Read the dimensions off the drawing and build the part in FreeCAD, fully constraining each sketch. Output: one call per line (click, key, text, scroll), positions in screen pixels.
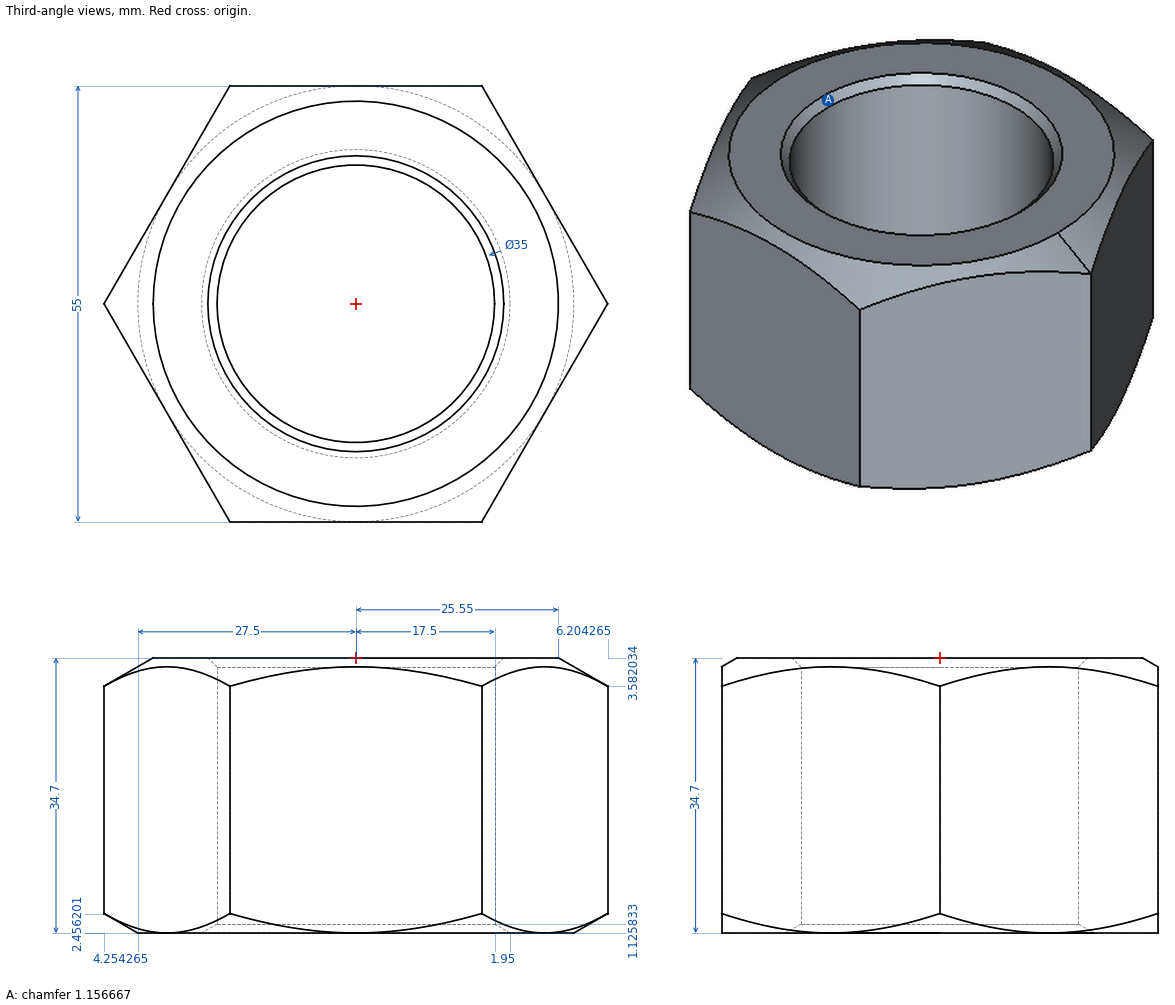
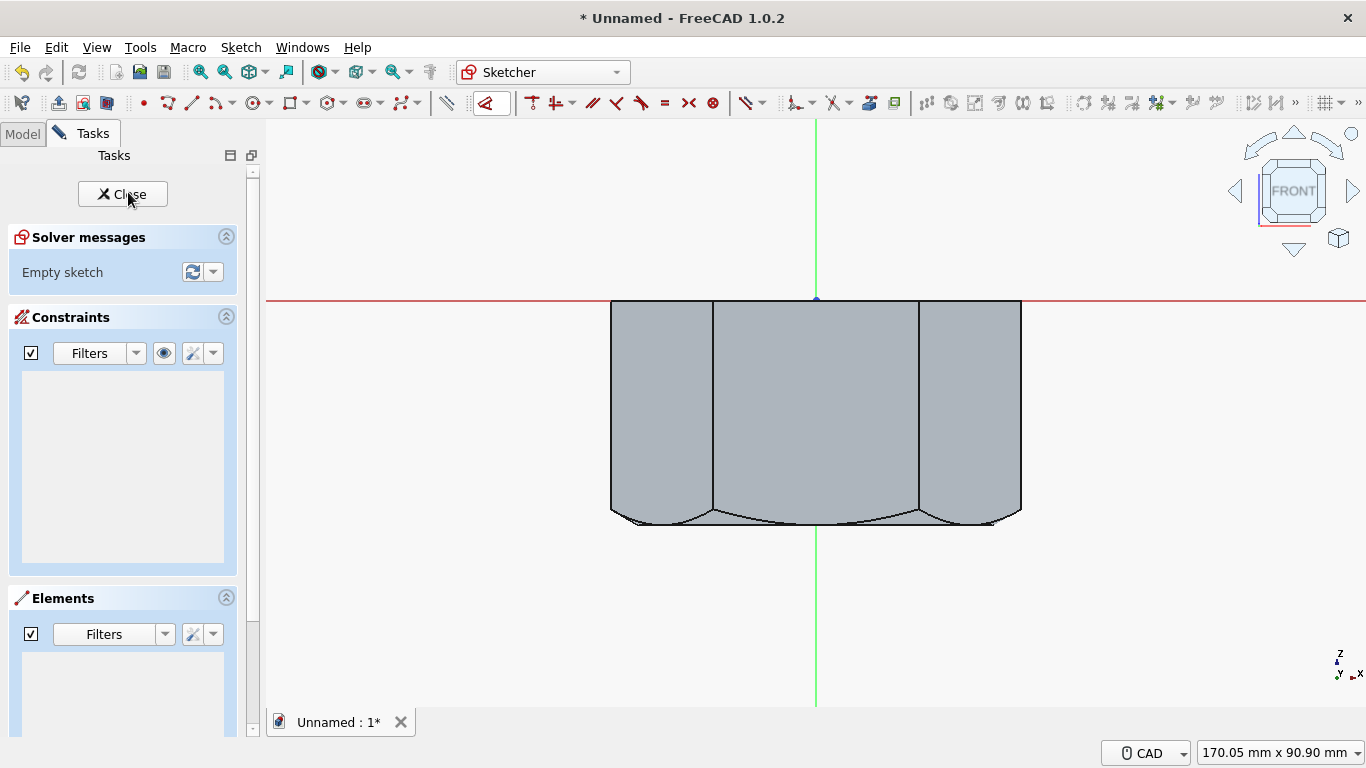
key(q)
key(s)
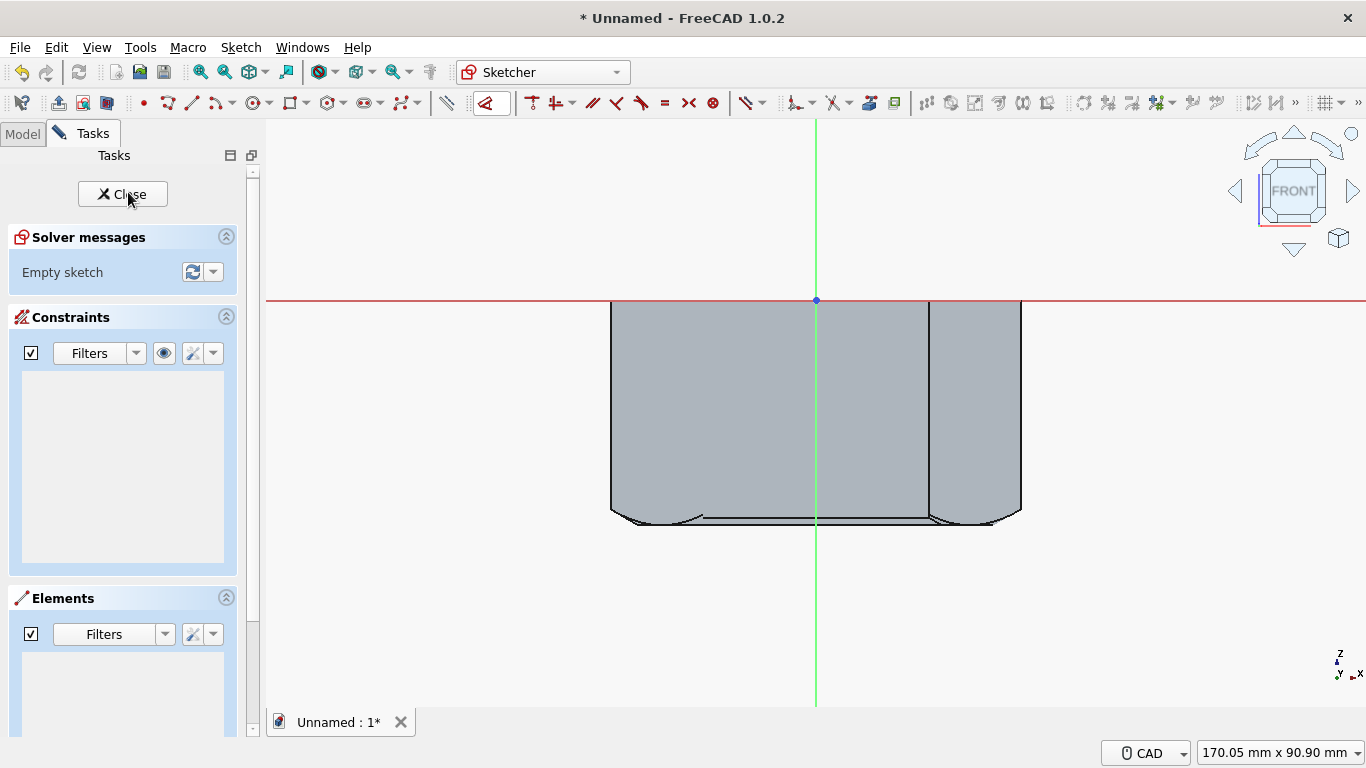
scroll(1018, 306, up, 14)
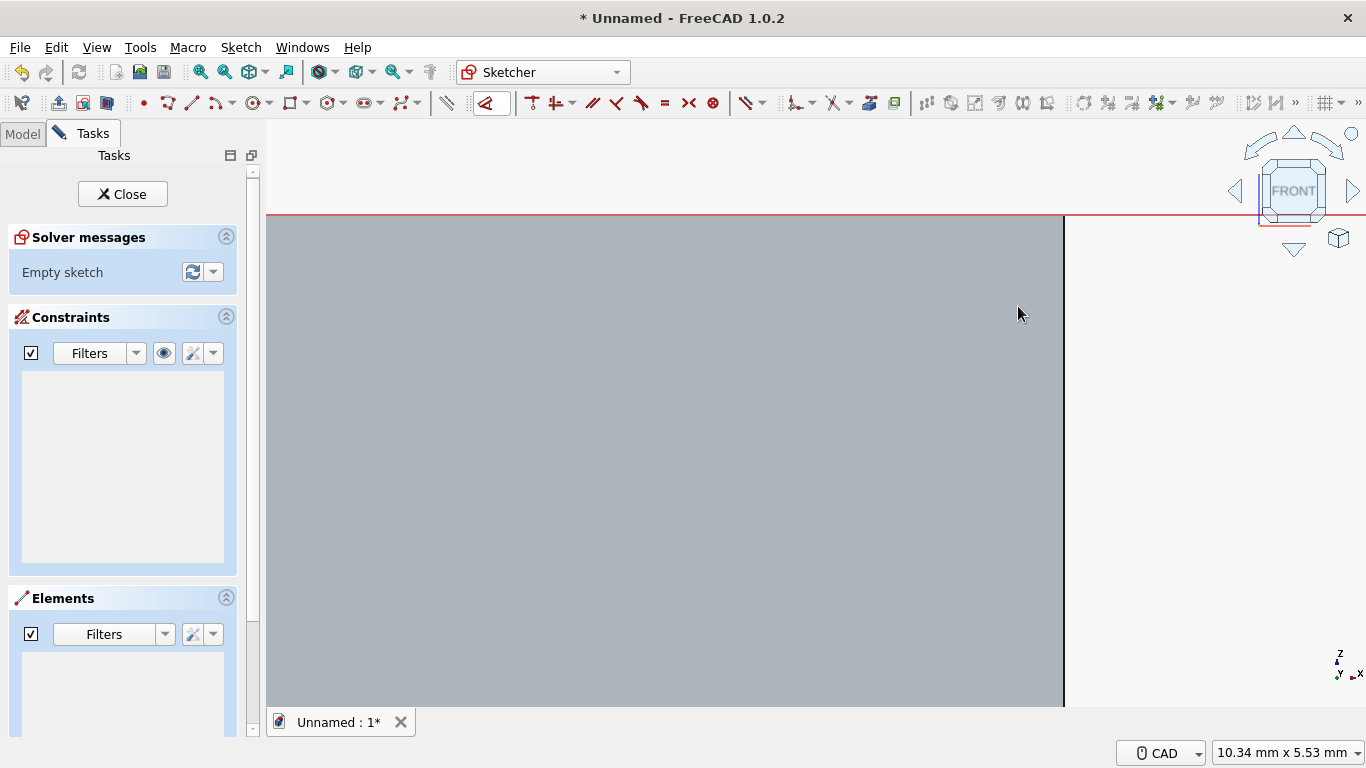
key(g)
key(m)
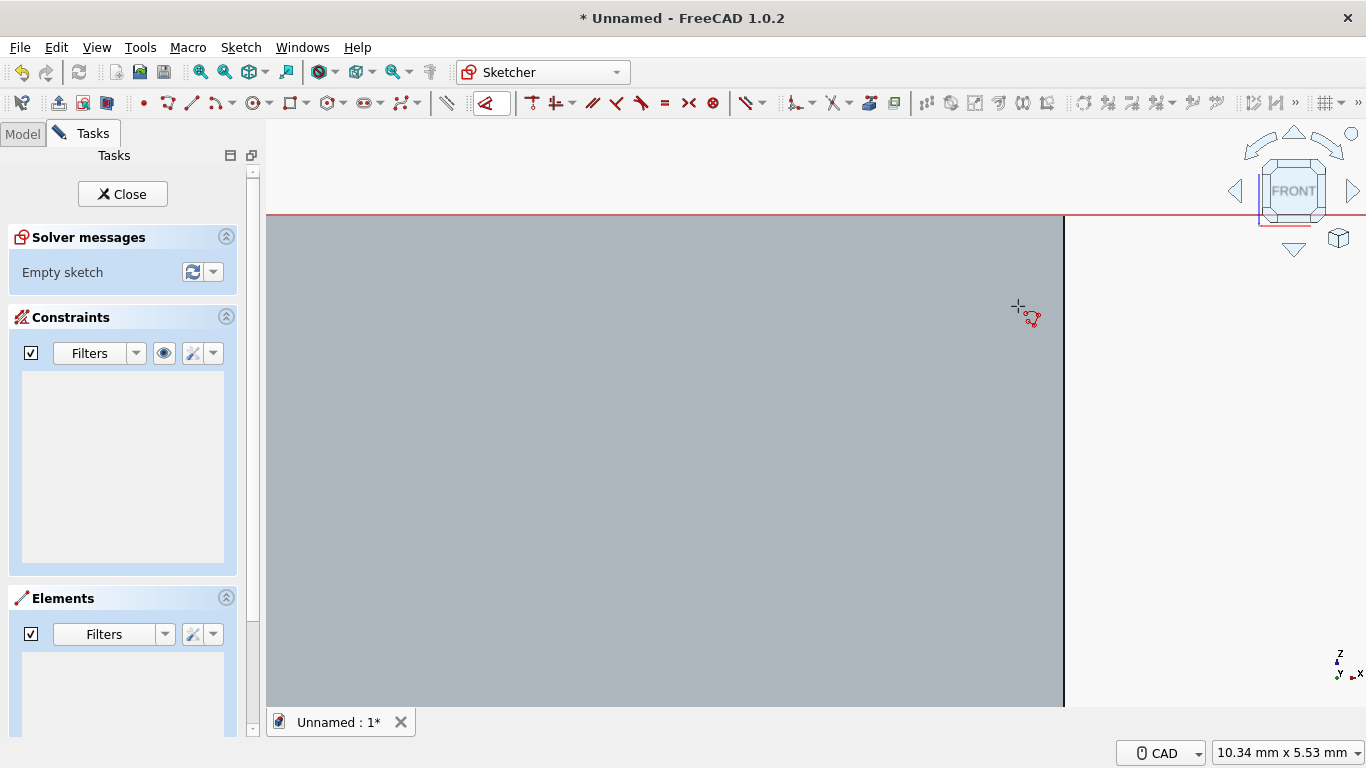
click(404, 215)
click(1064, 224)
click(1064, 596)
click(404, 215)
key(Escape)
key(Escape)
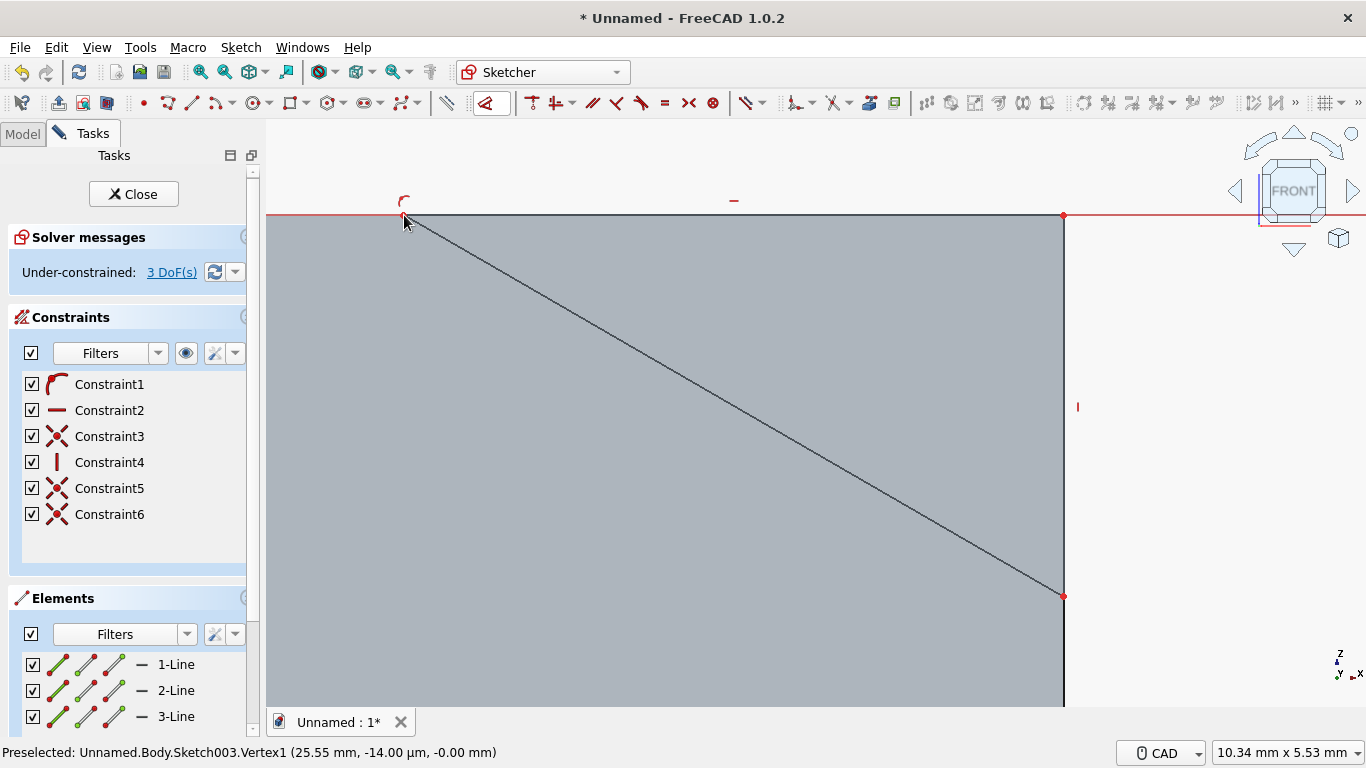
click(404, 215)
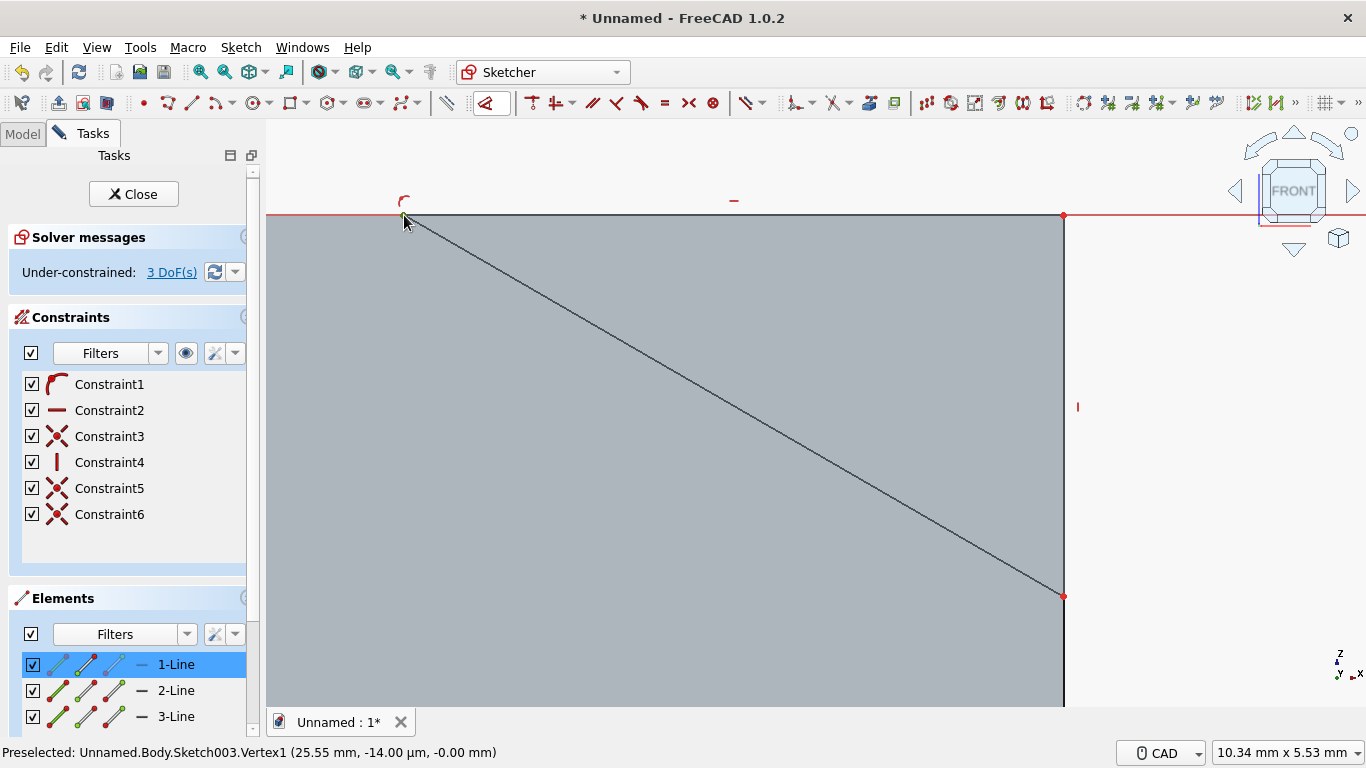
key(l)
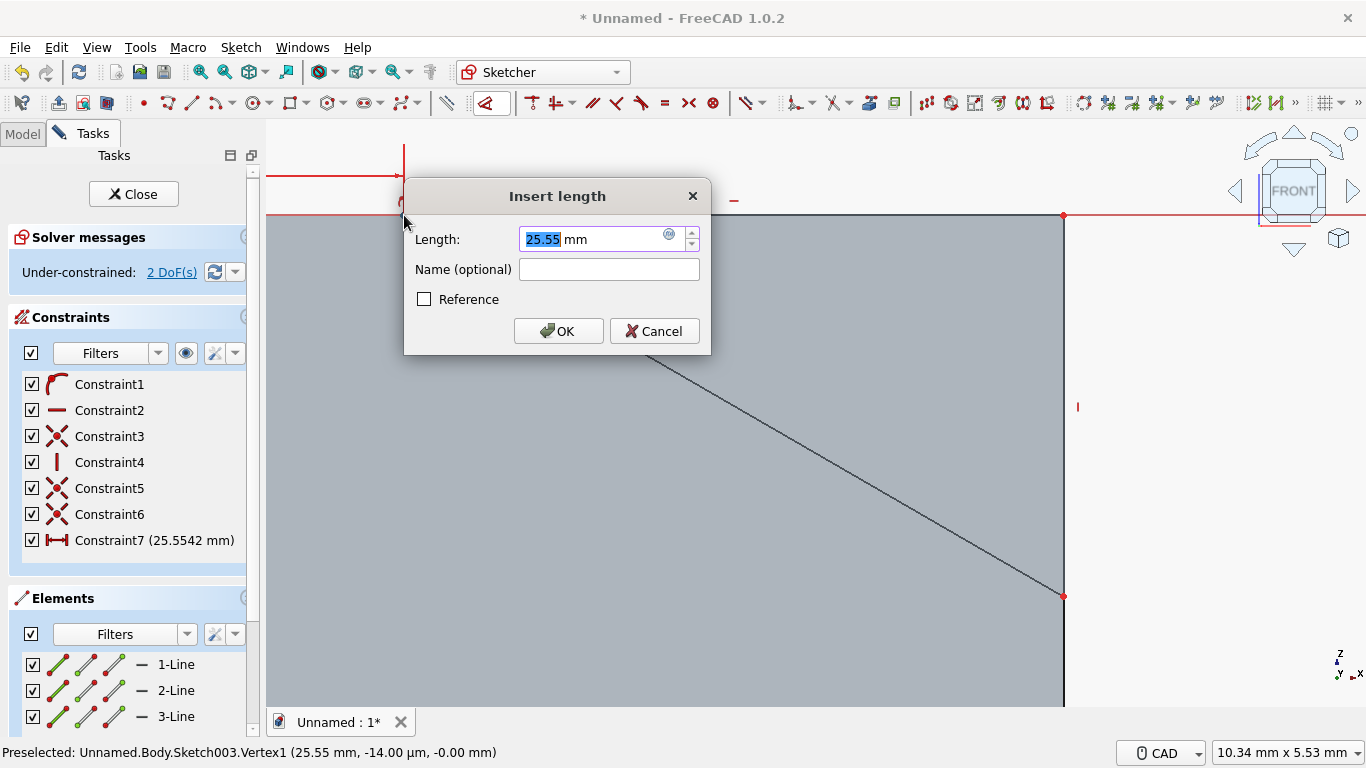
text(25.55)
key(Return)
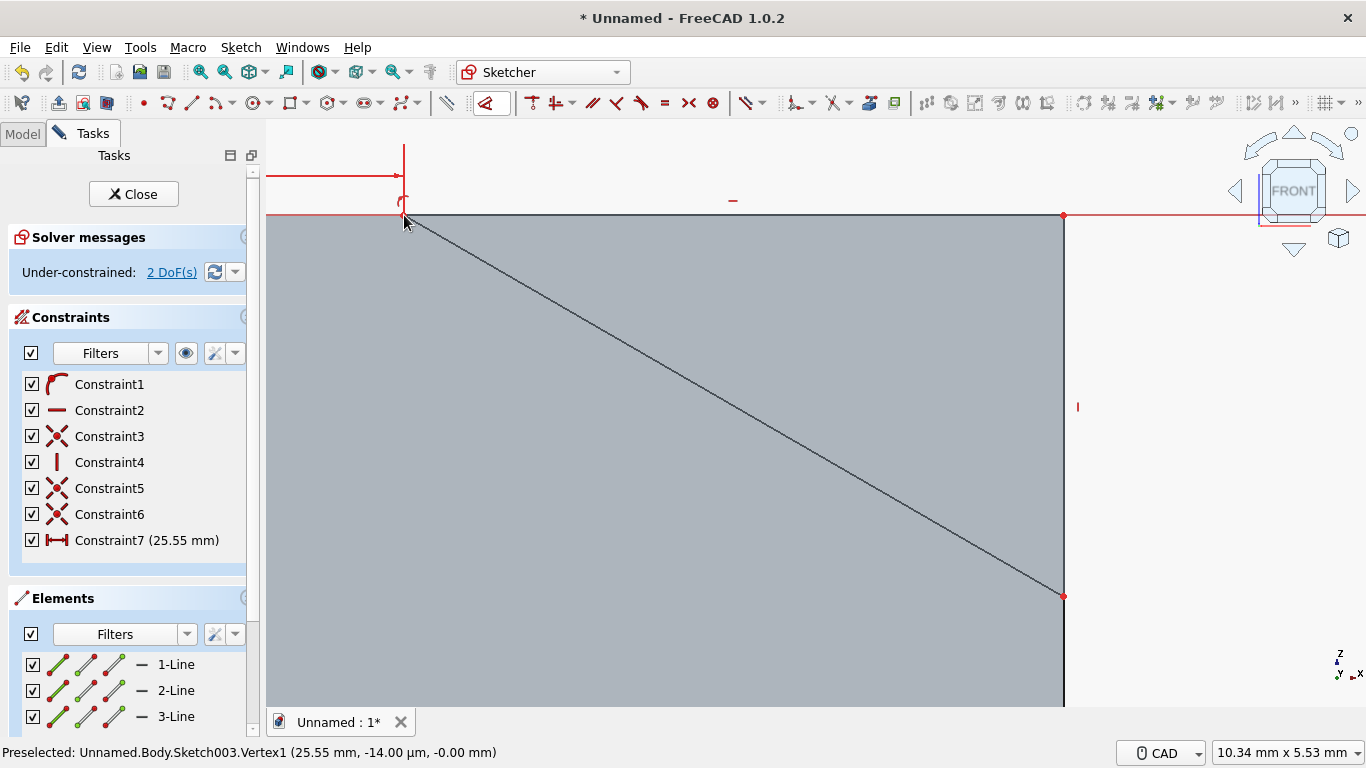
click(602, 215)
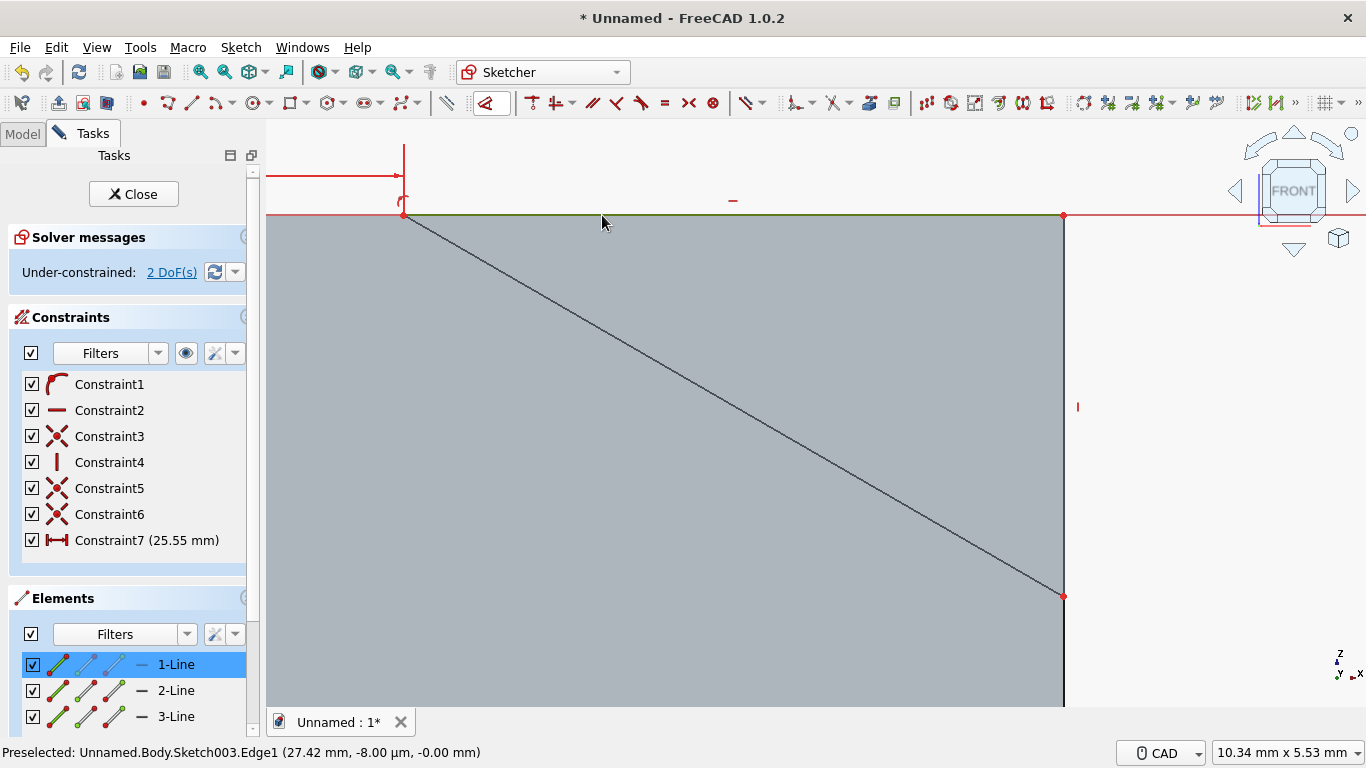
key(l)